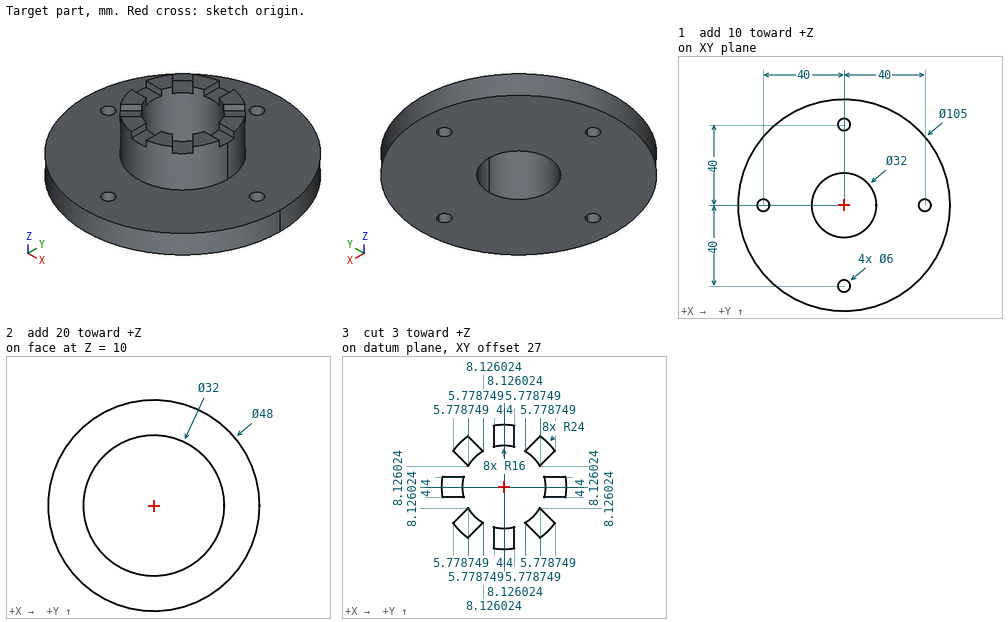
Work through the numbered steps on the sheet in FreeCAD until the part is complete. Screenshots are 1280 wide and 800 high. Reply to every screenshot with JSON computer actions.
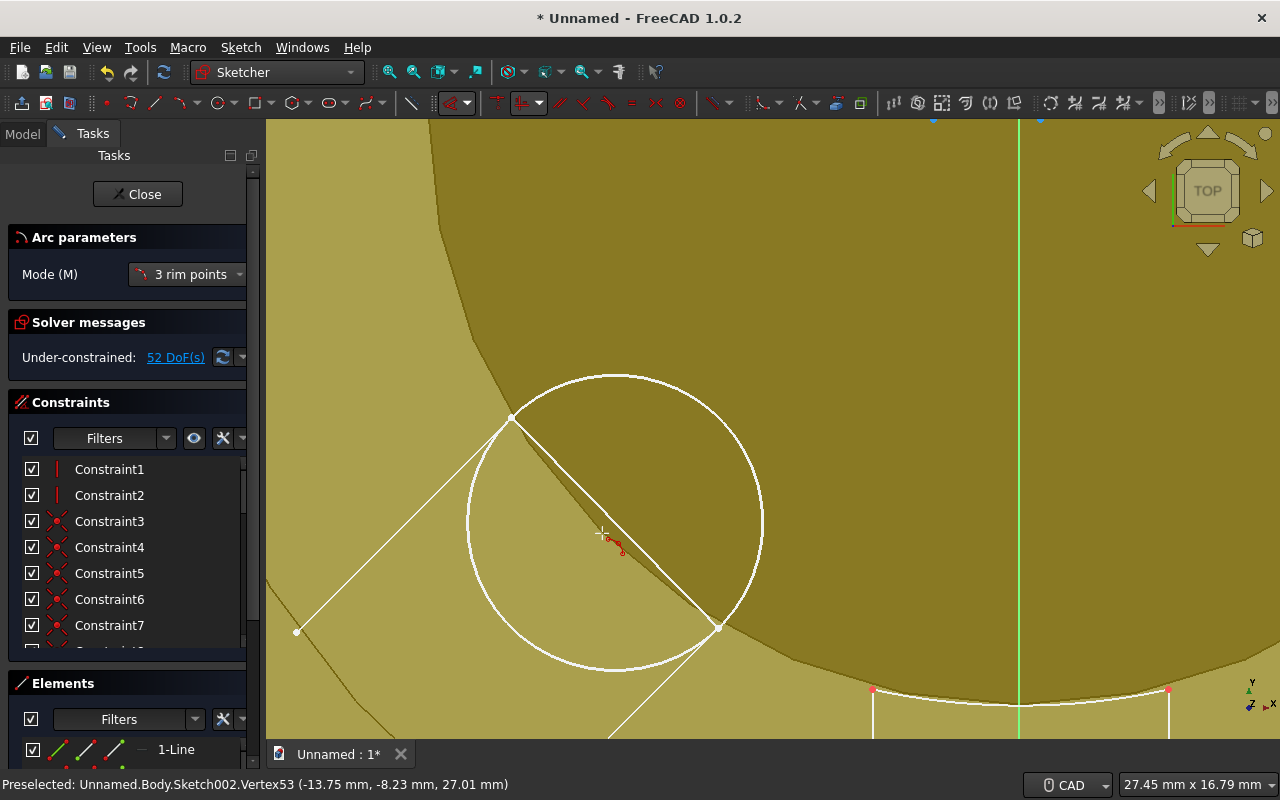
{"action": "left_click", "coordinate": [602, 531]}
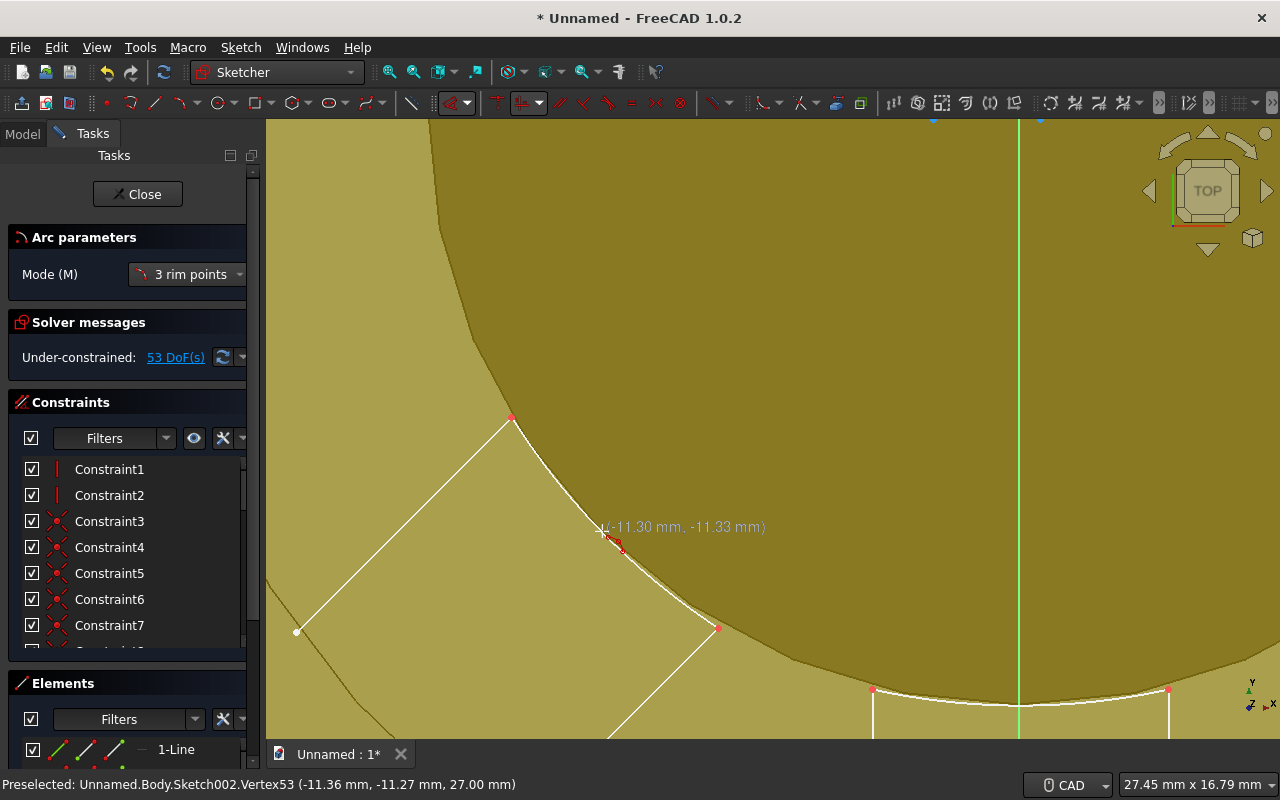
{"action": "scroll", "coordinate": [601, 532], "scroll_direction": "down", "scroll_amount": 7}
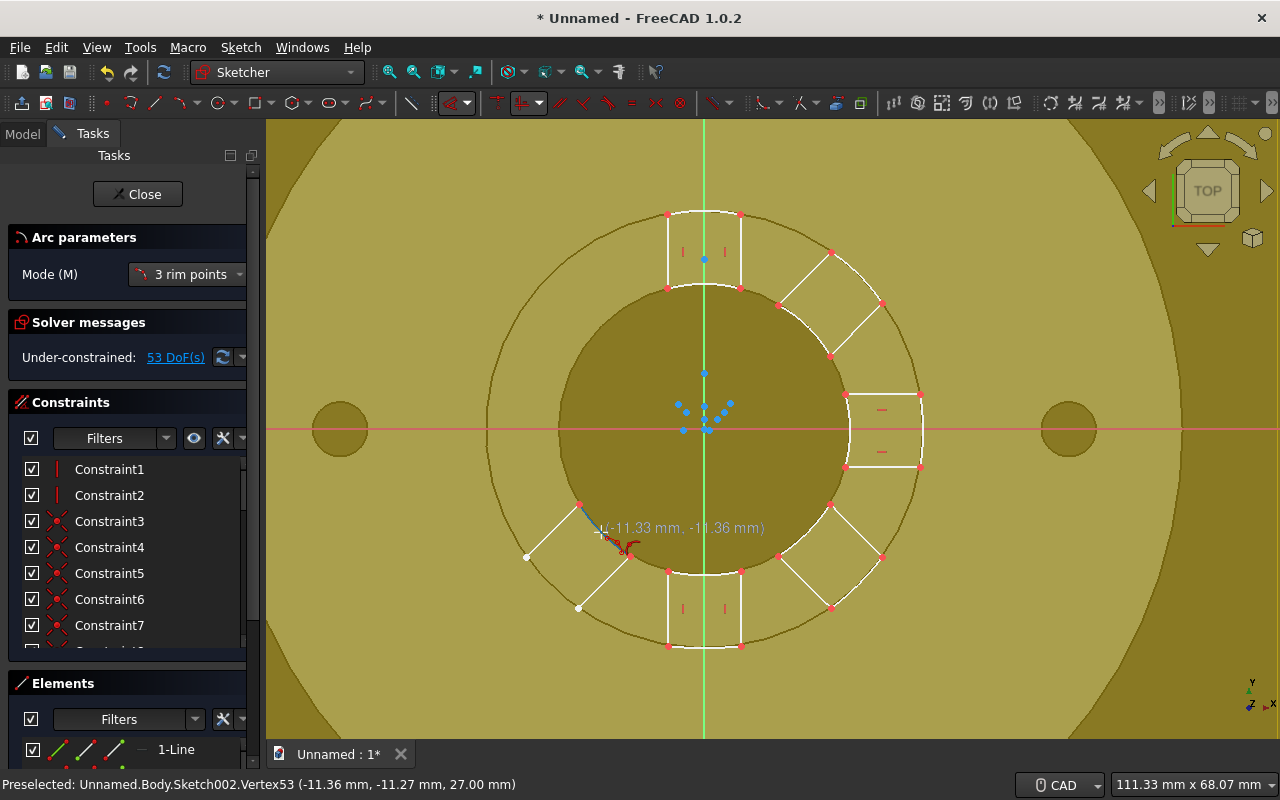
{"action": "left_click", "coordinate": [526, 557]}
{"action": "left_click", "coordinate": [578, 608]}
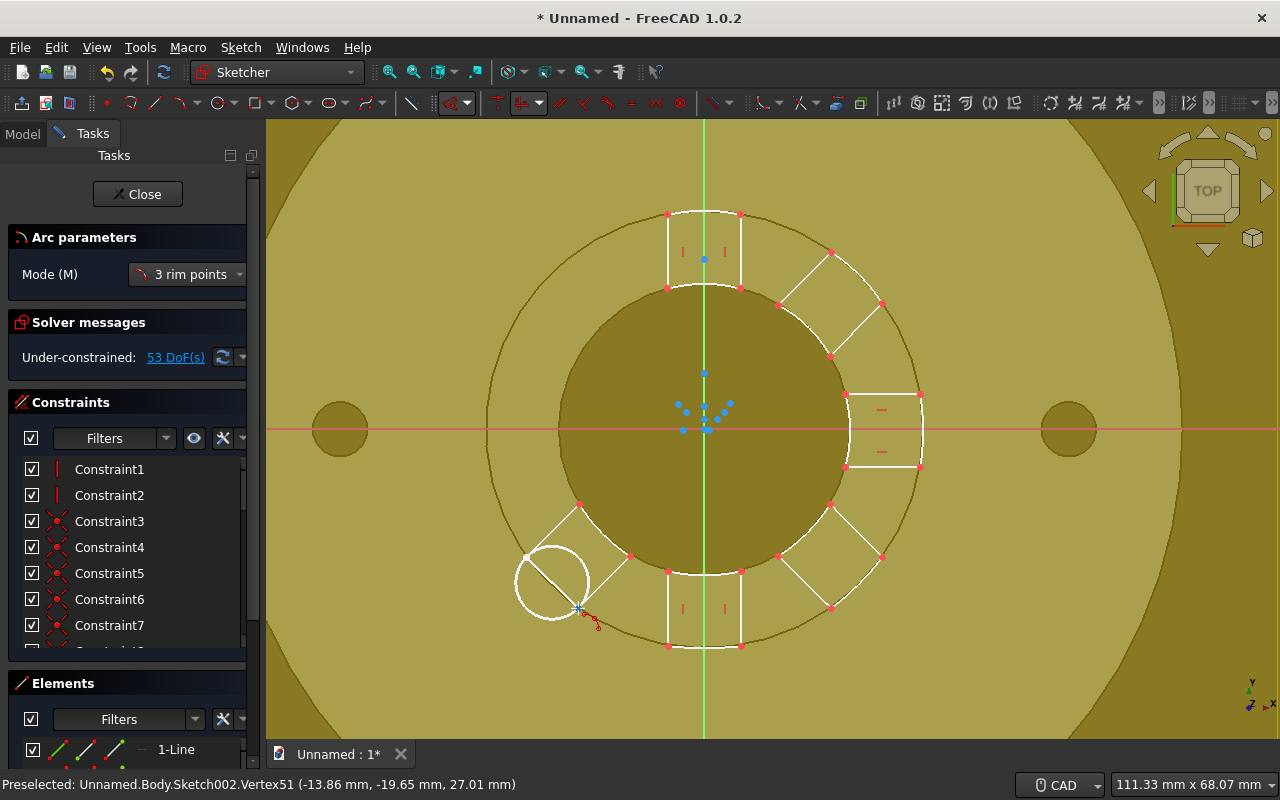
{"action": "scroll", "coordinate": [550, 584], "scroll_direction": "up", "scroll_amount": 9}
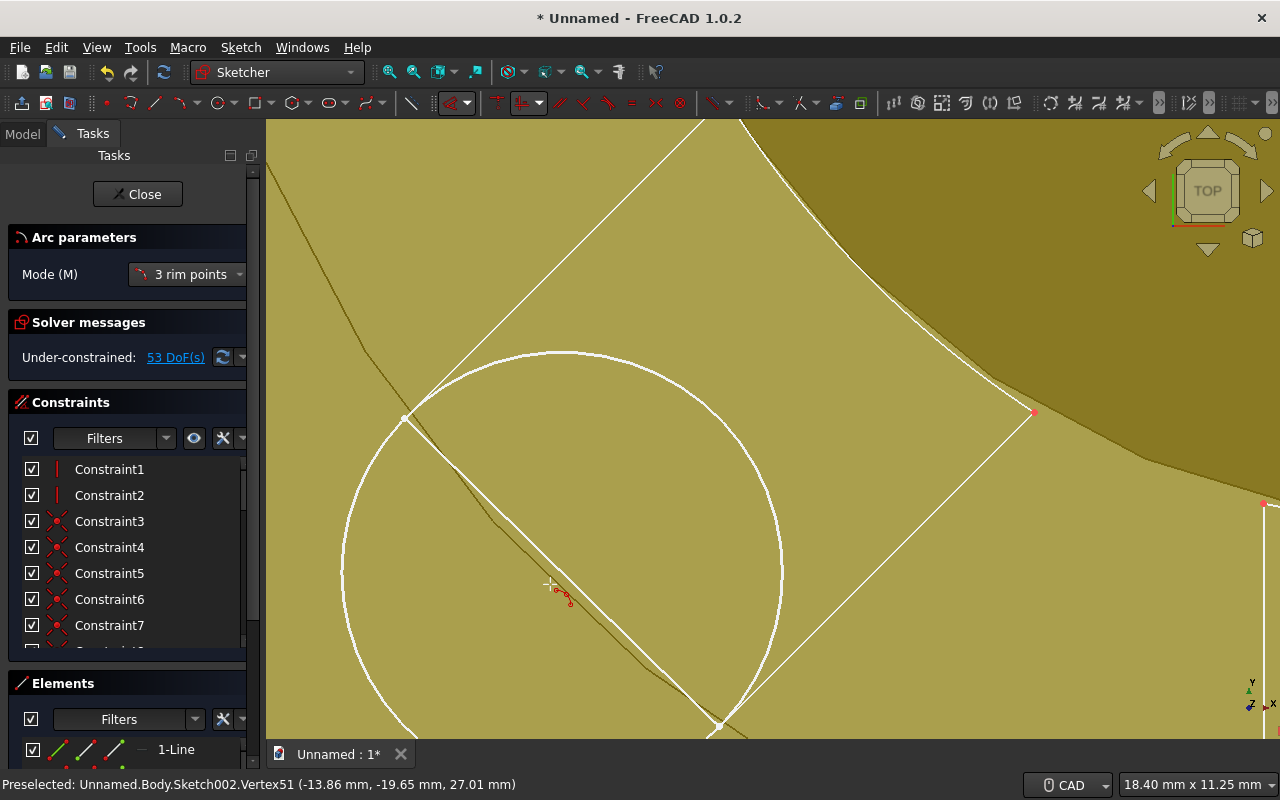
{"action": "left_click", "coordinate": [548, 579]}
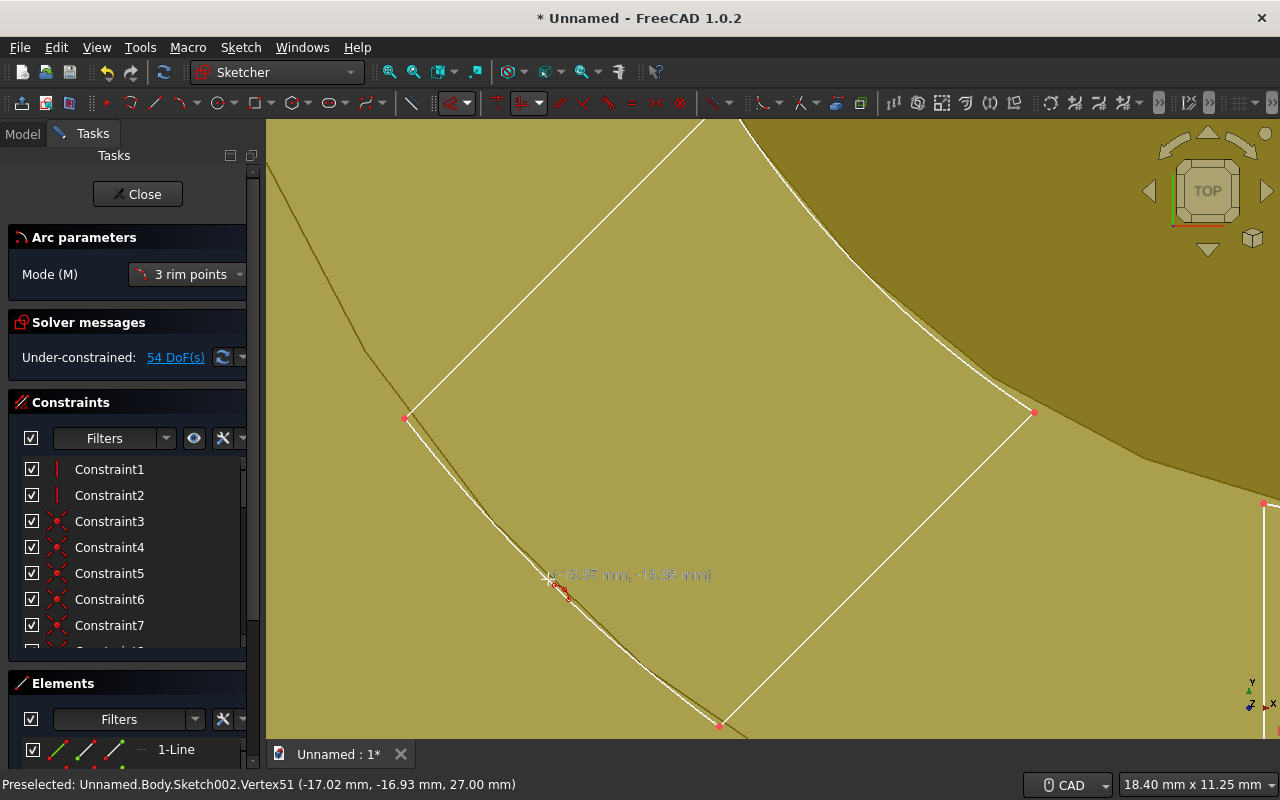
{"action": "left_click", "coordinate": [156, 104]}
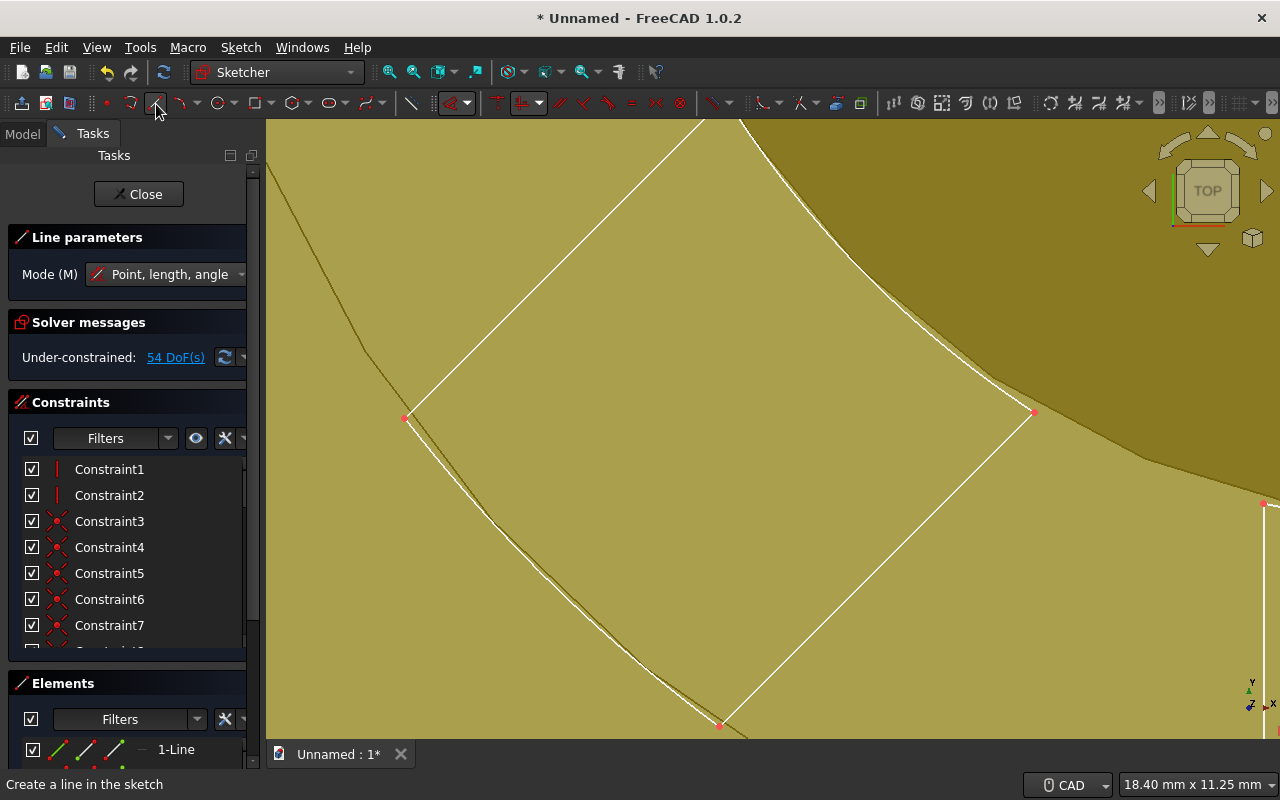
{"action": "scroll", "coordinate": [550, 584], "scroll_direction": "down", "scroll_amount": 9}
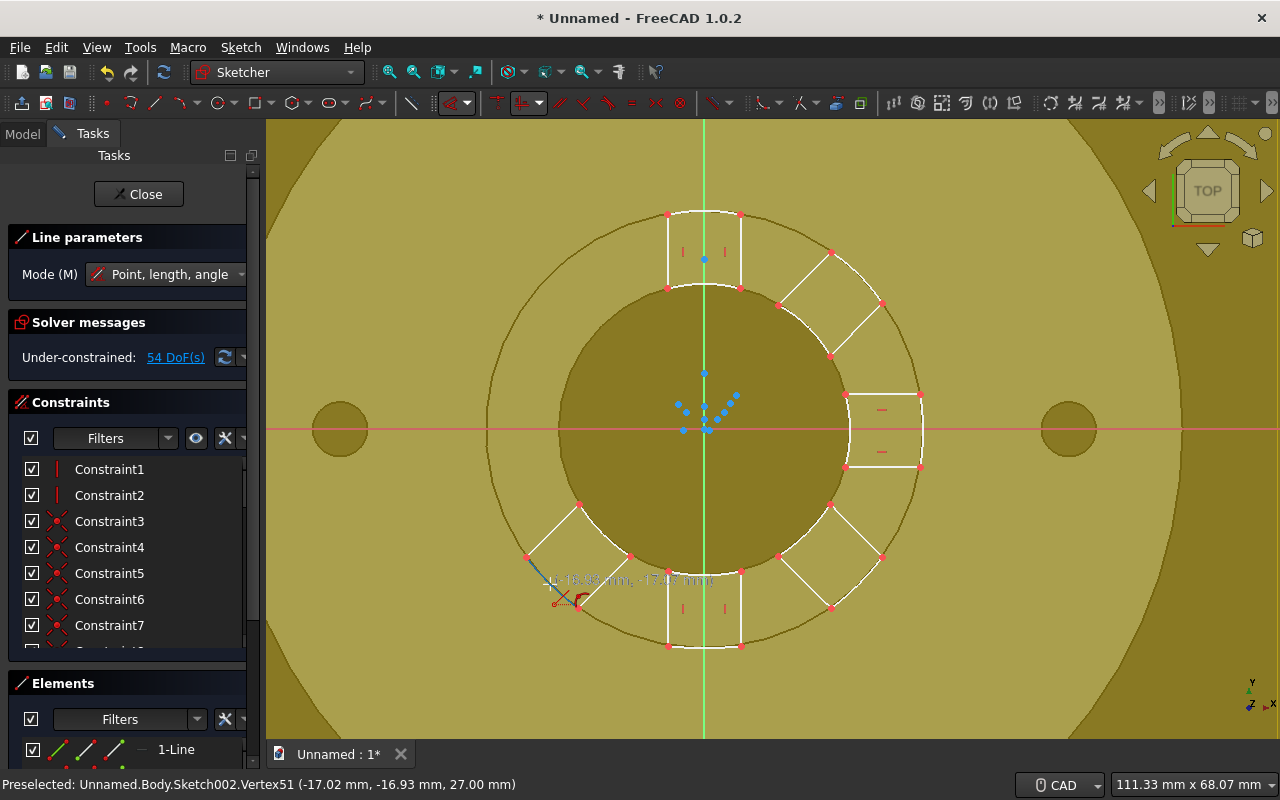
{"action": "left_click", "coordinate": [489, 466]}
{"action": "left_click", "coordinate": [563, 466]}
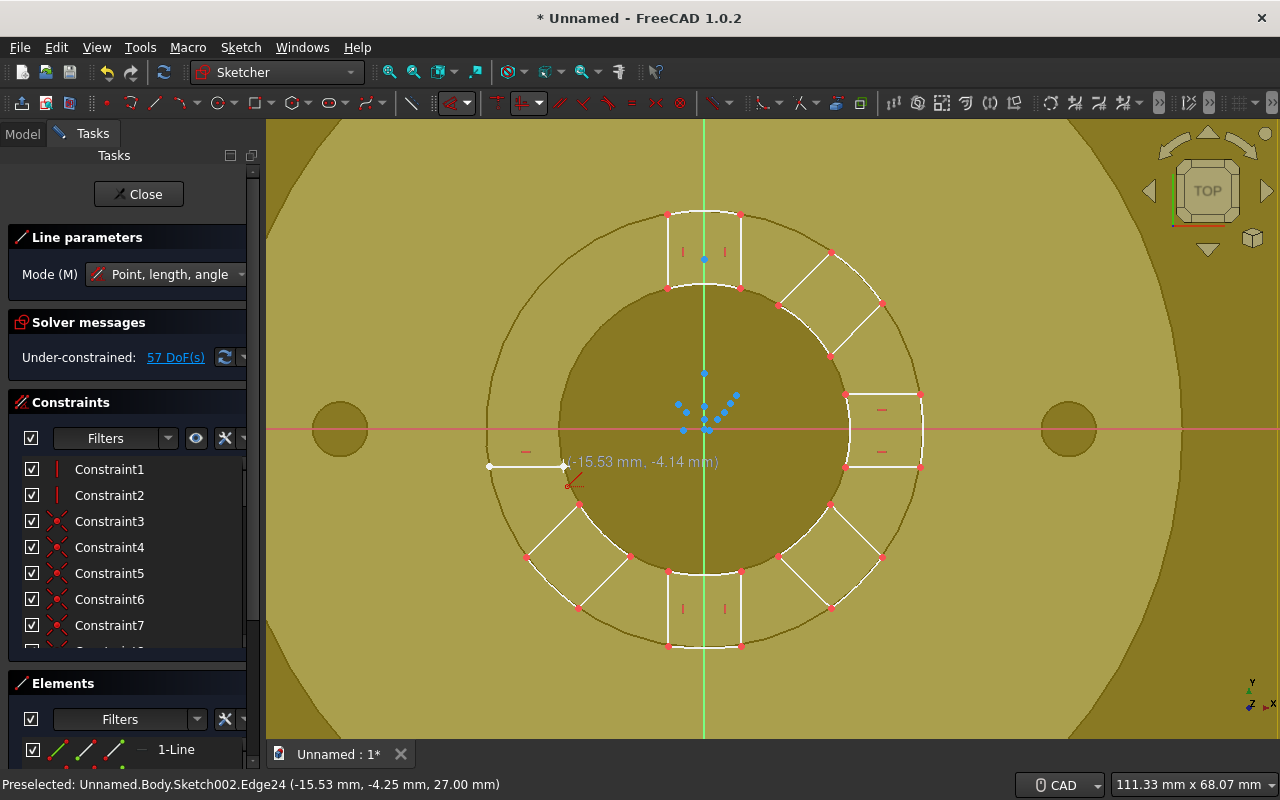
{"action": "left_click", "coordinate": [563, 393]}
{"action": "left_click", "coordinate": [489, 393]}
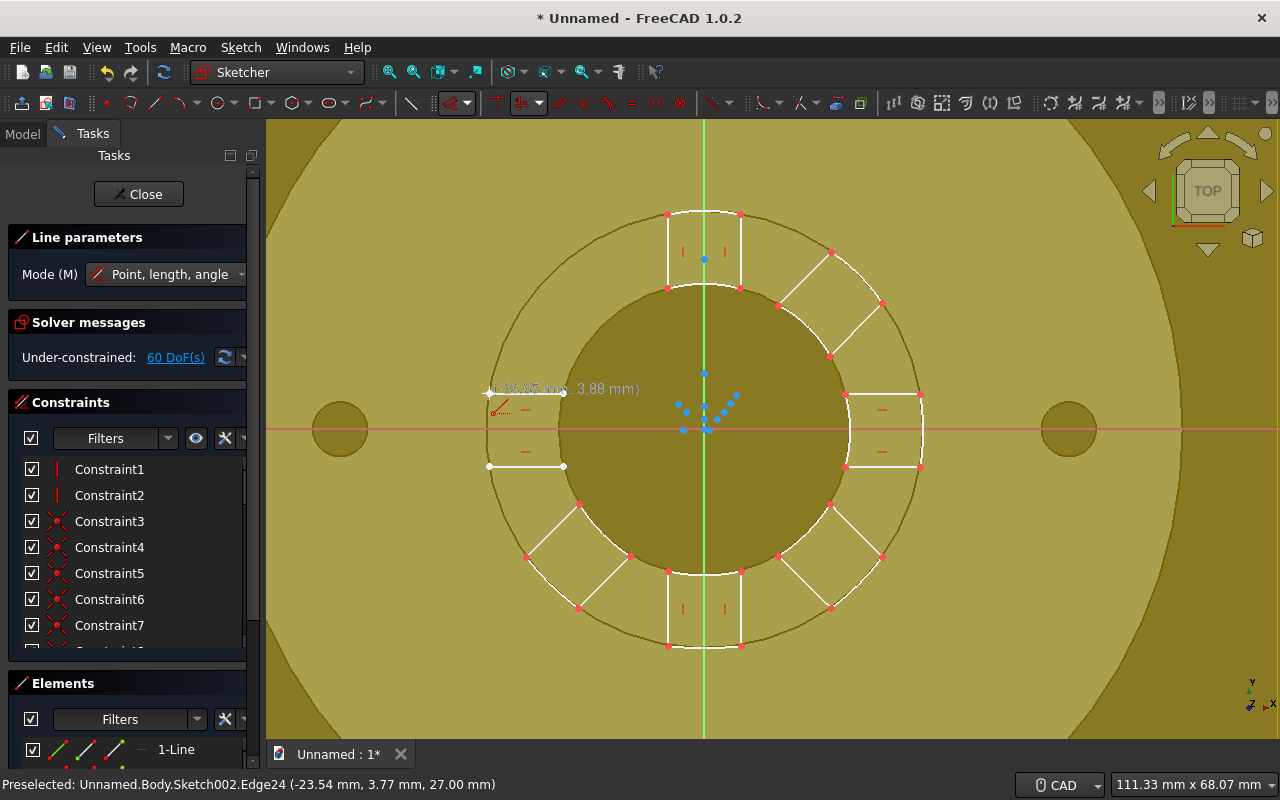
{"action": "left_click", "coordinate": [180, 104]}